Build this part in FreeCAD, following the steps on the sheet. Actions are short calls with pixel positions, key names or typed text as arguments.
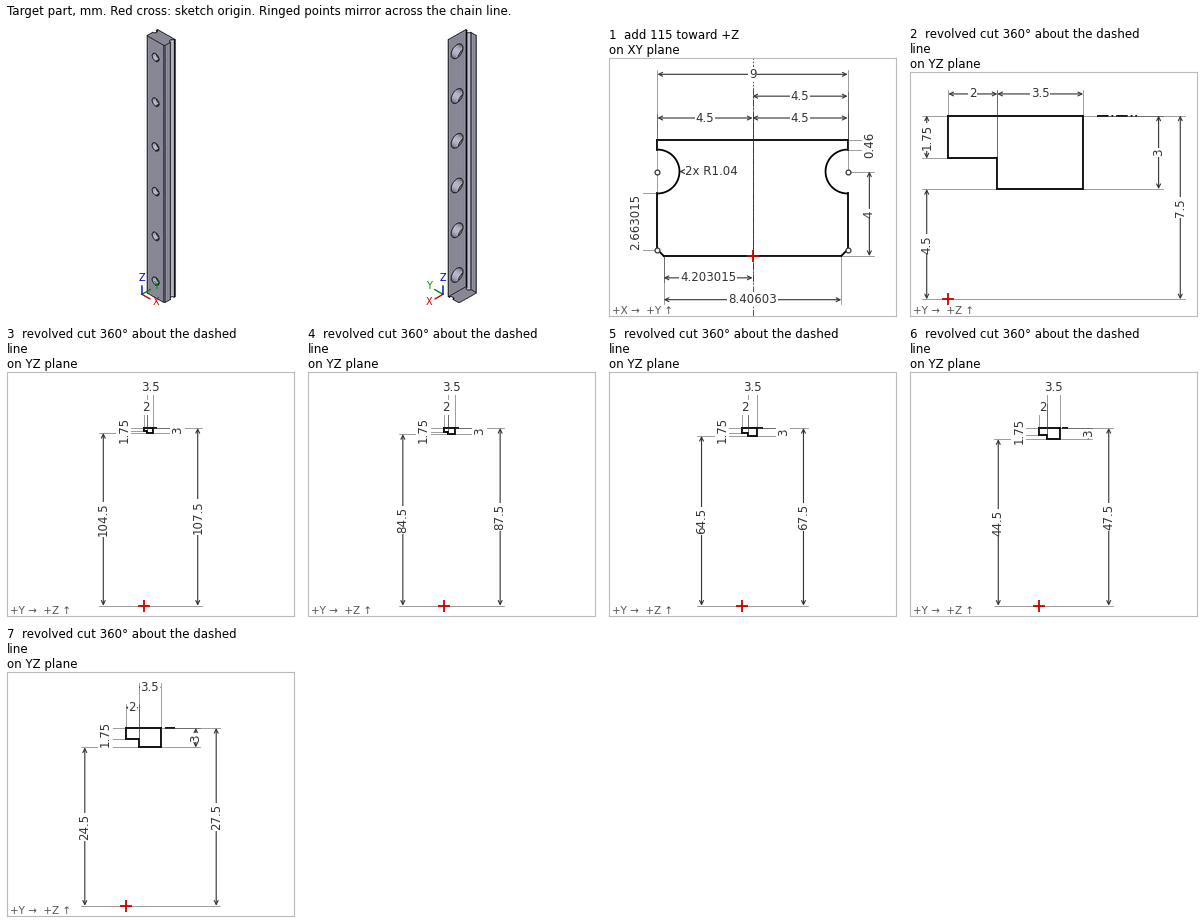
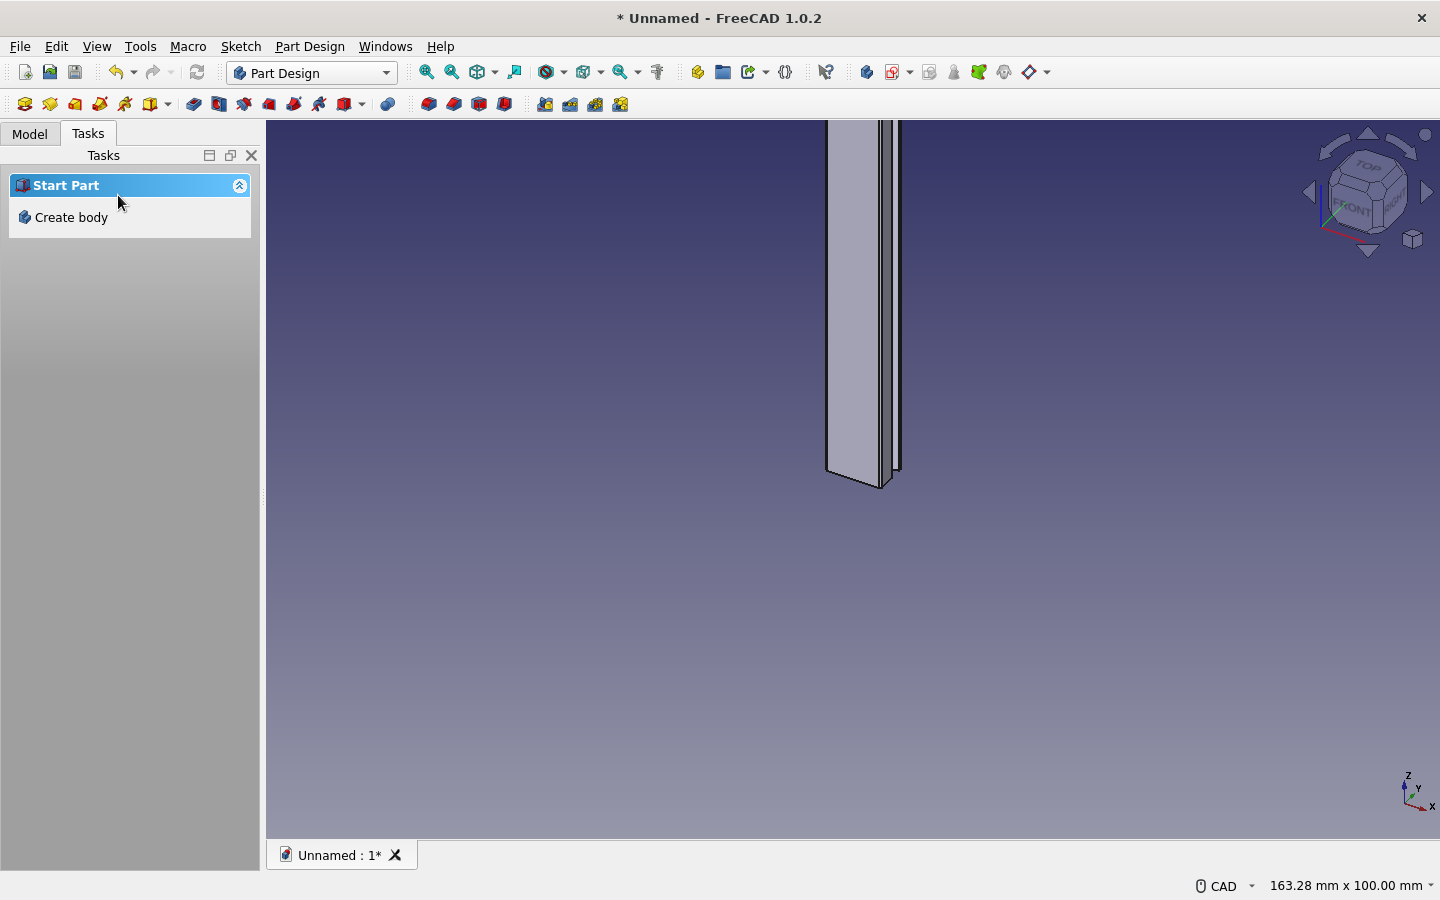
key(v)
key(f)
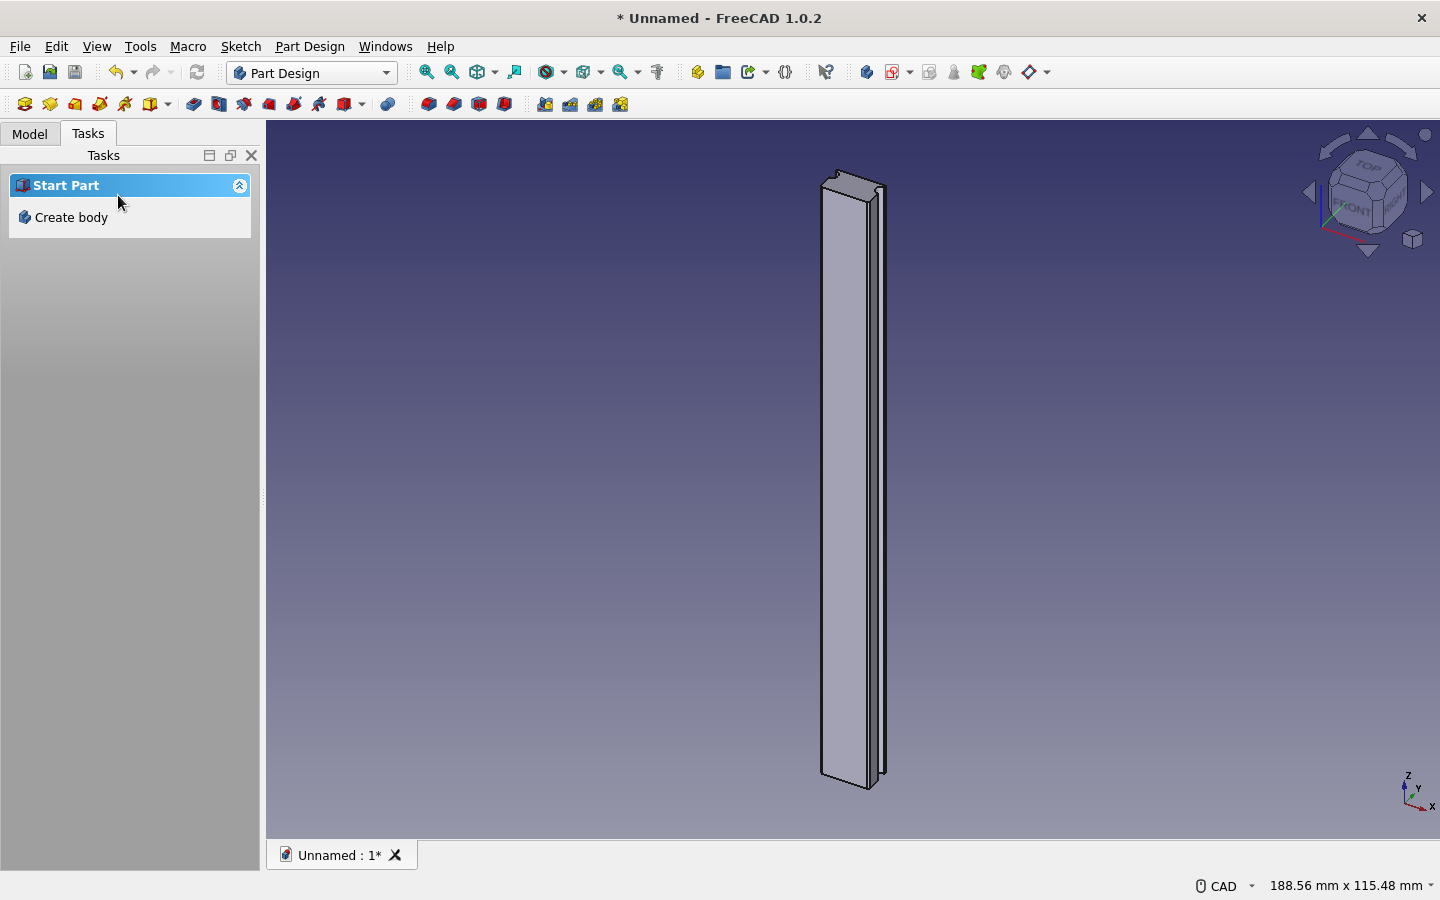
click(892, 72)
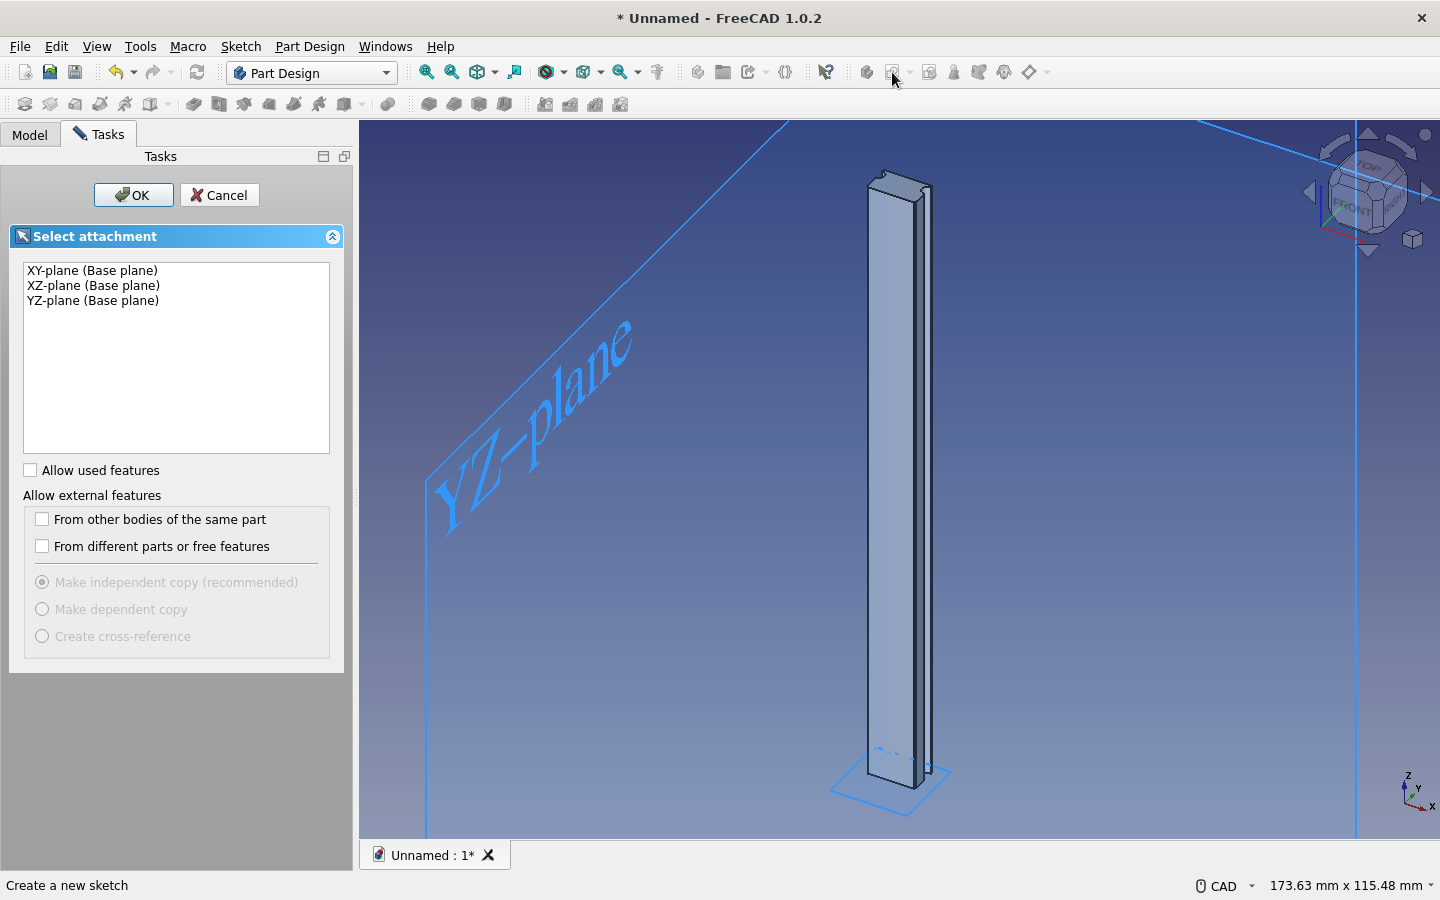
click(84, 300)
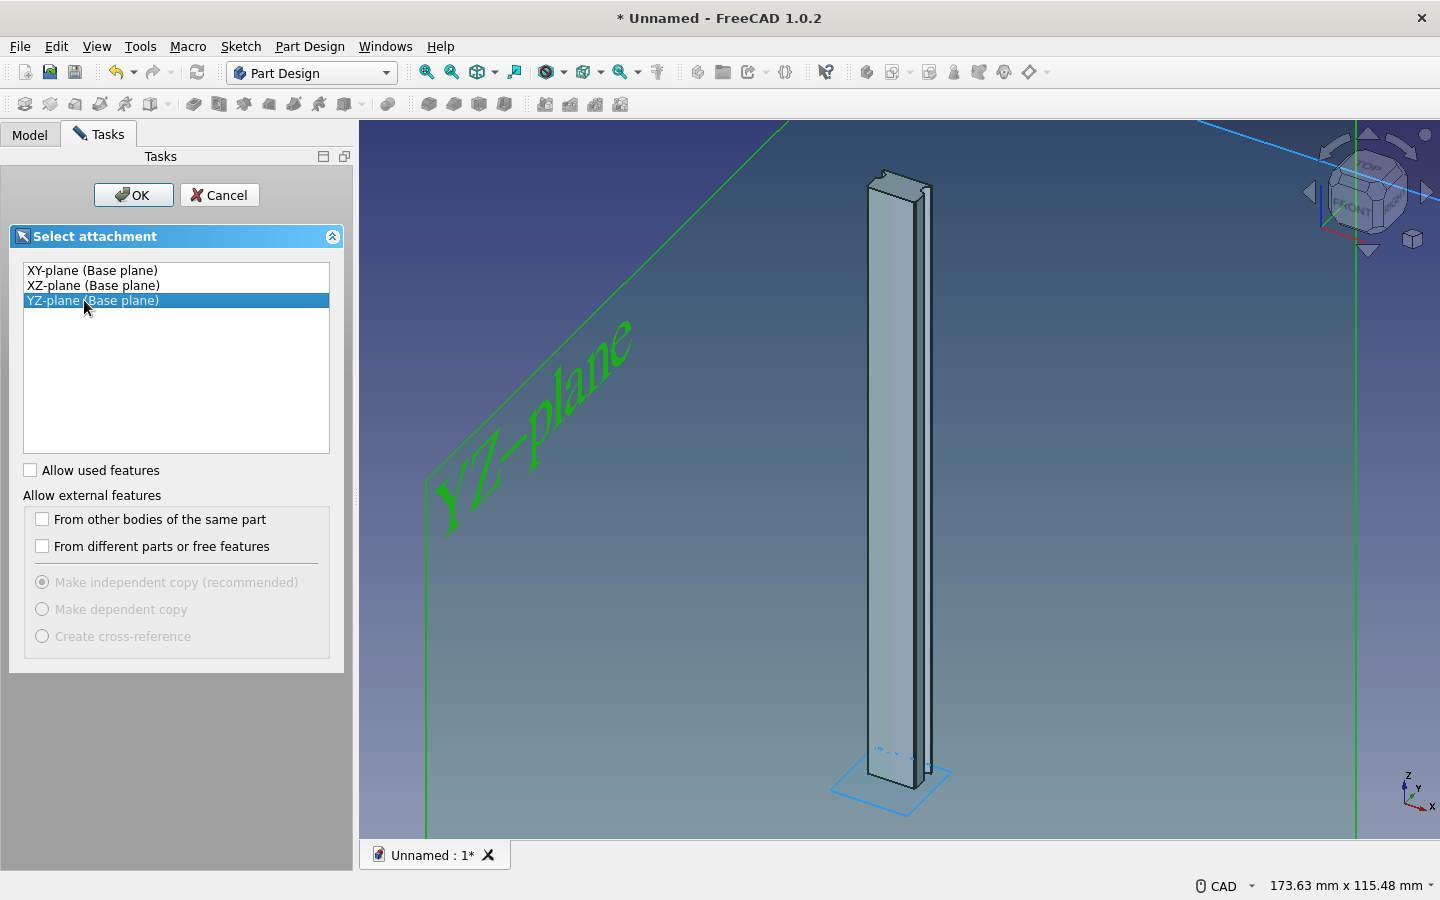
click(134, 195)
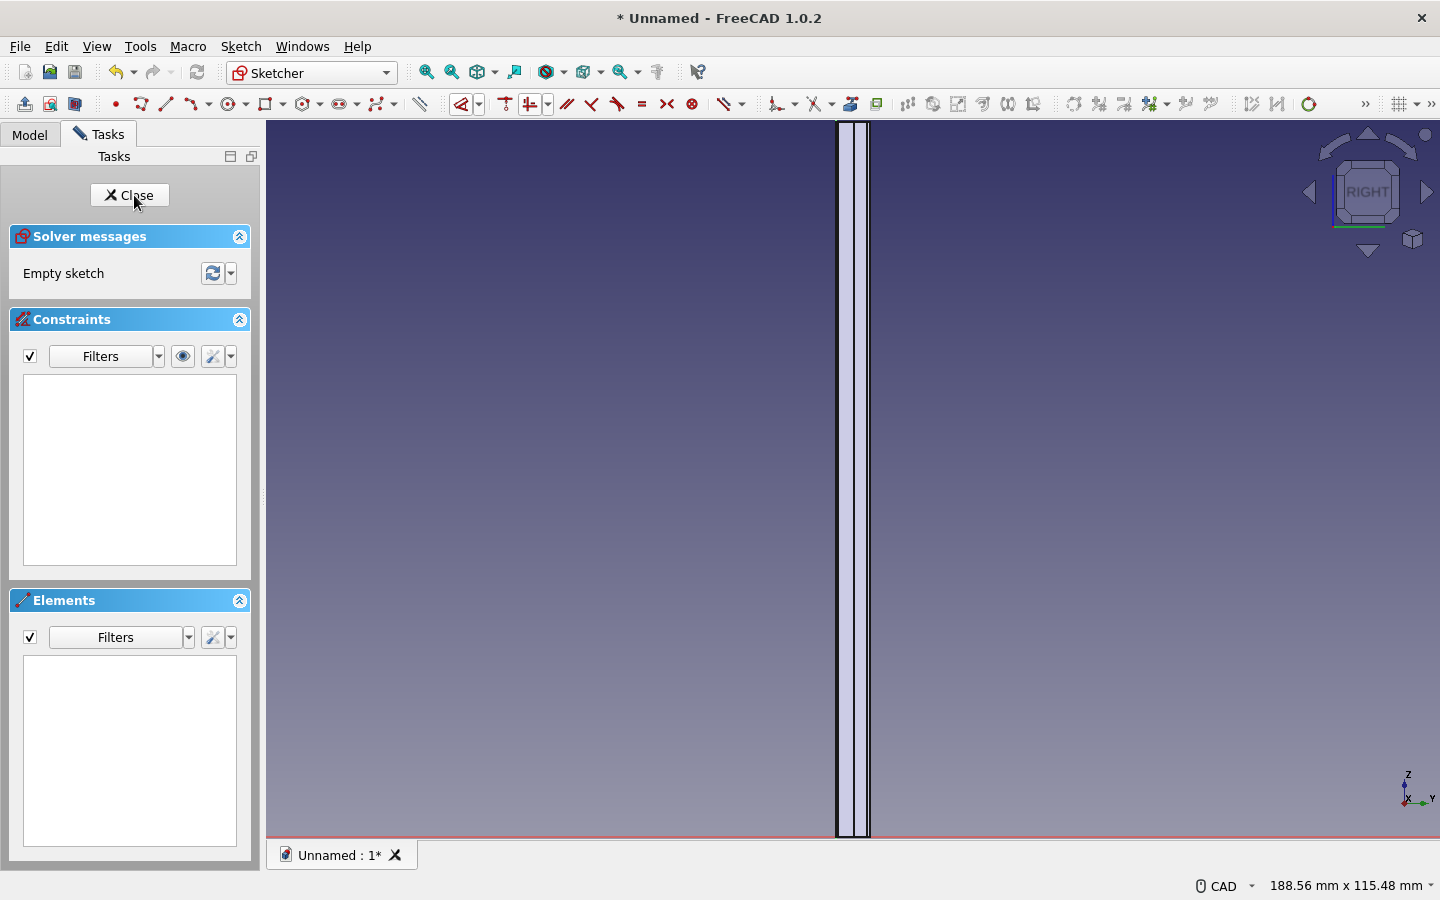
click(75, 104)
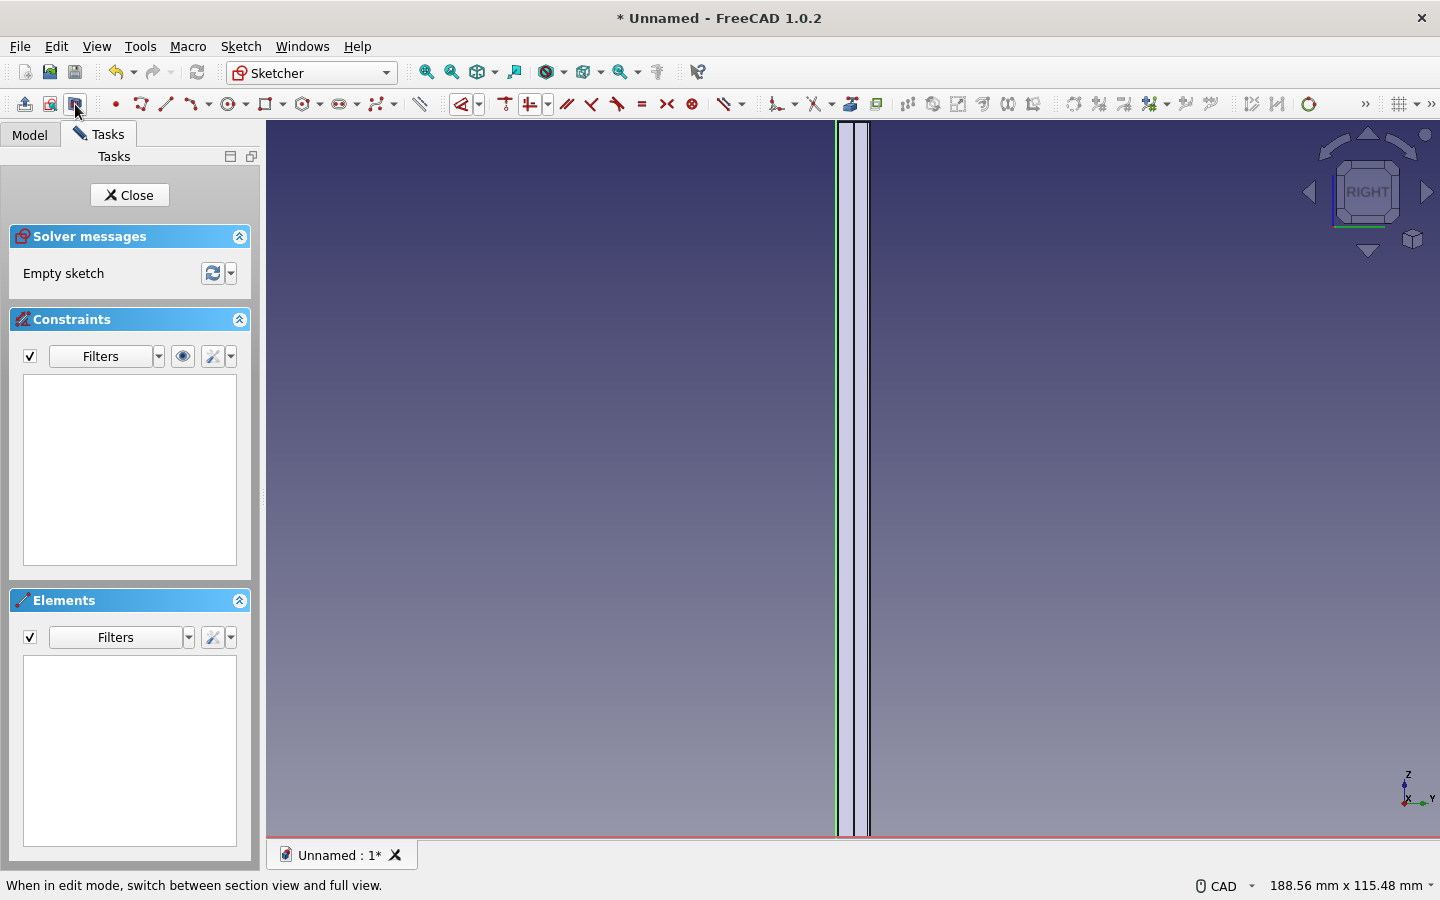
scroll(784, 480, down, 5)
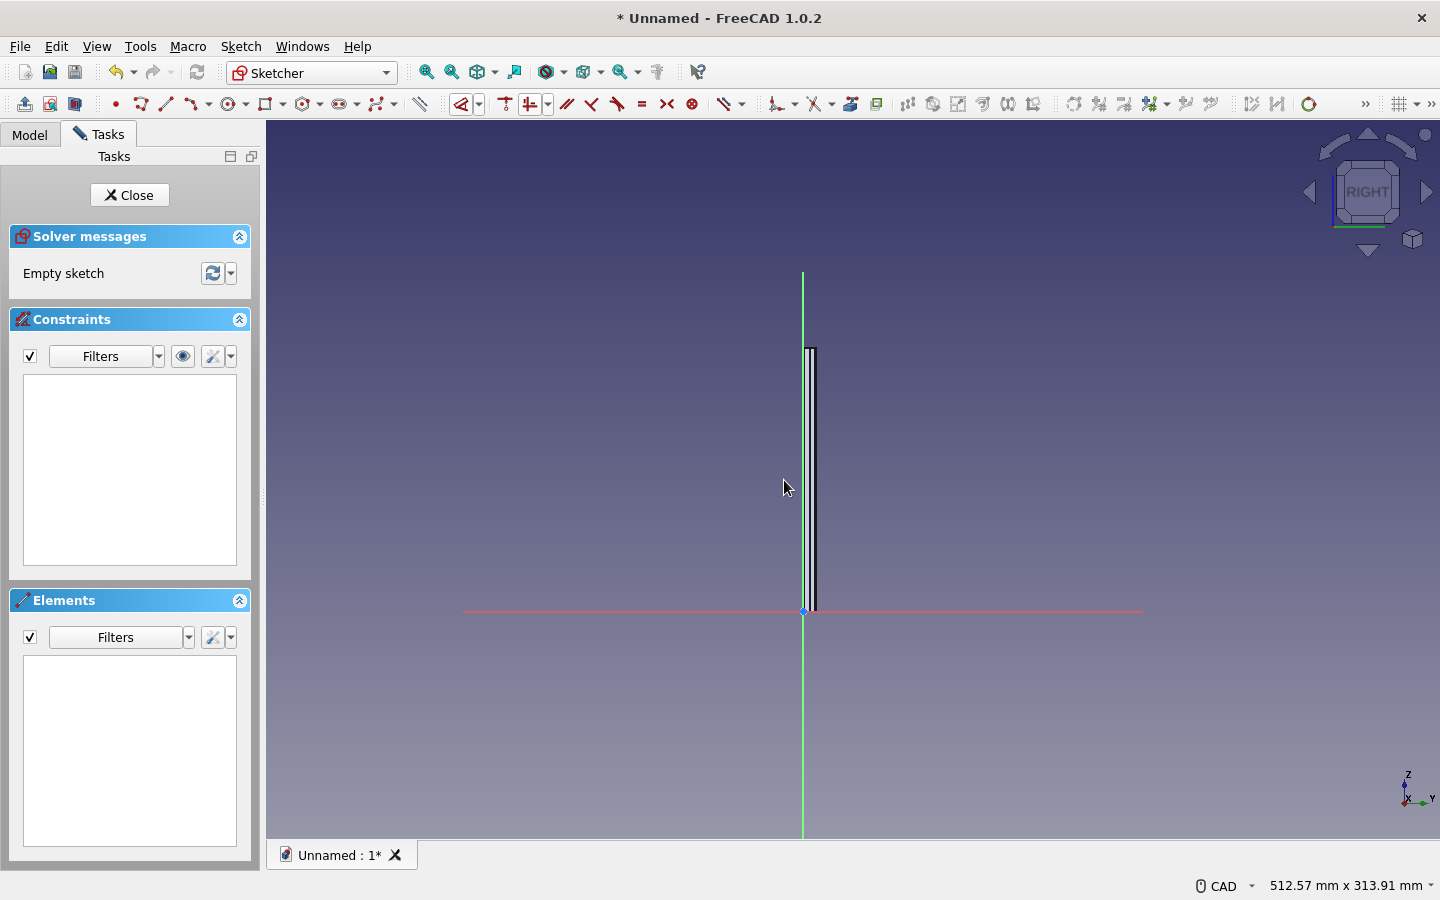
scroll(814, 610, up, 15)